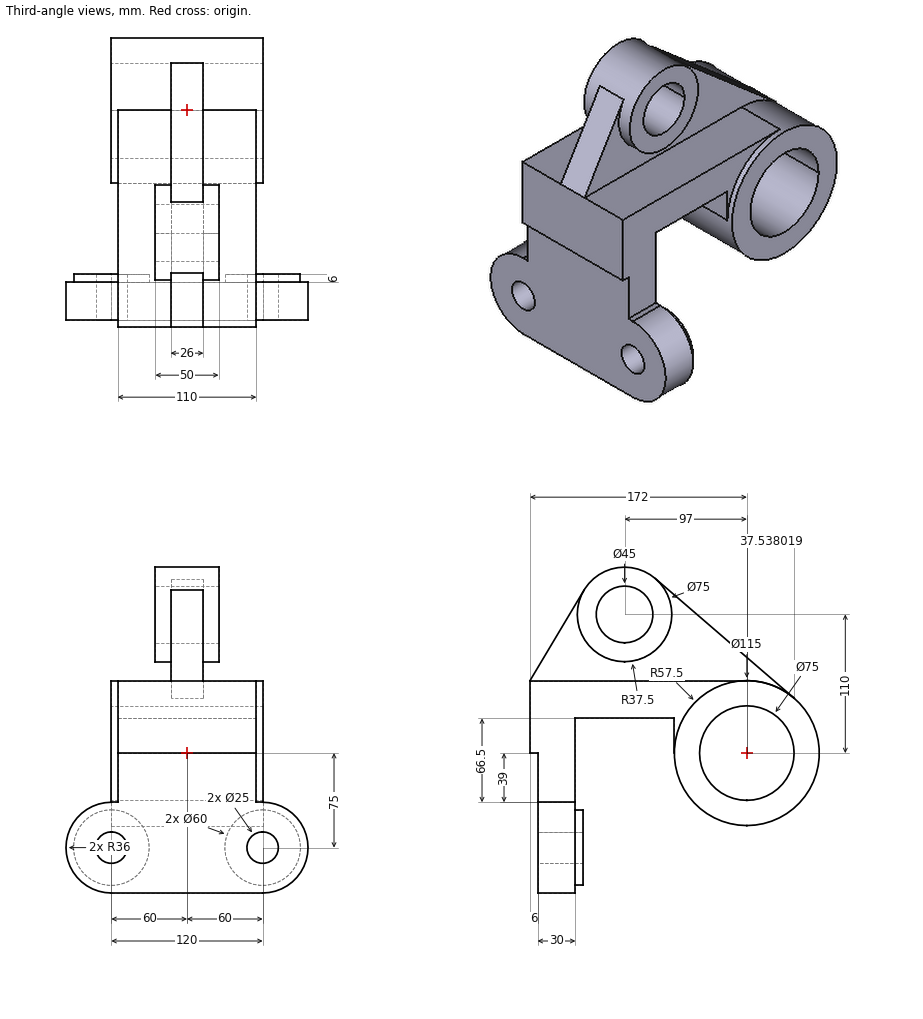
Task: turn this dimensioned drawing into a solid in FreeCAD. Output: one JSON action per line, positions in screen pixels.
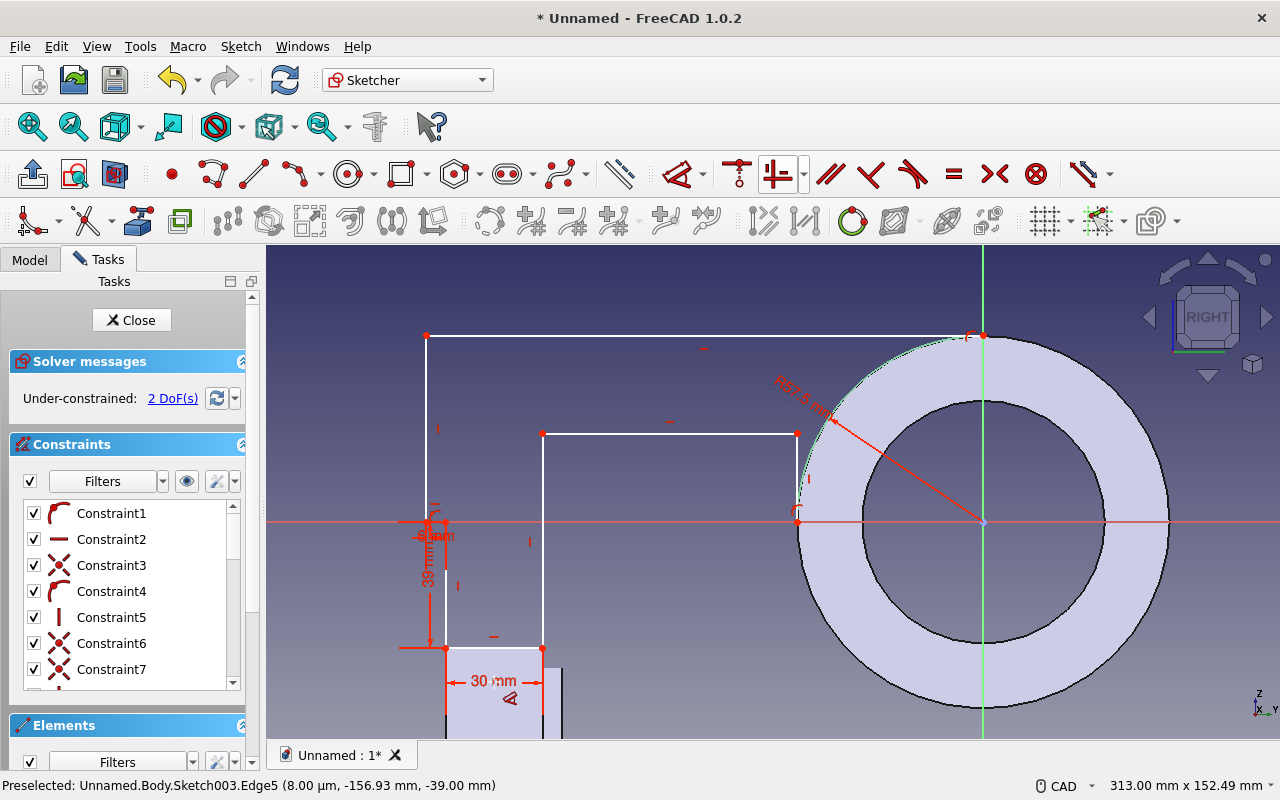
{"action": "left_click", "coordinate": [816, 336]}
{"action": "left_click", "coordinate": [705, 302]}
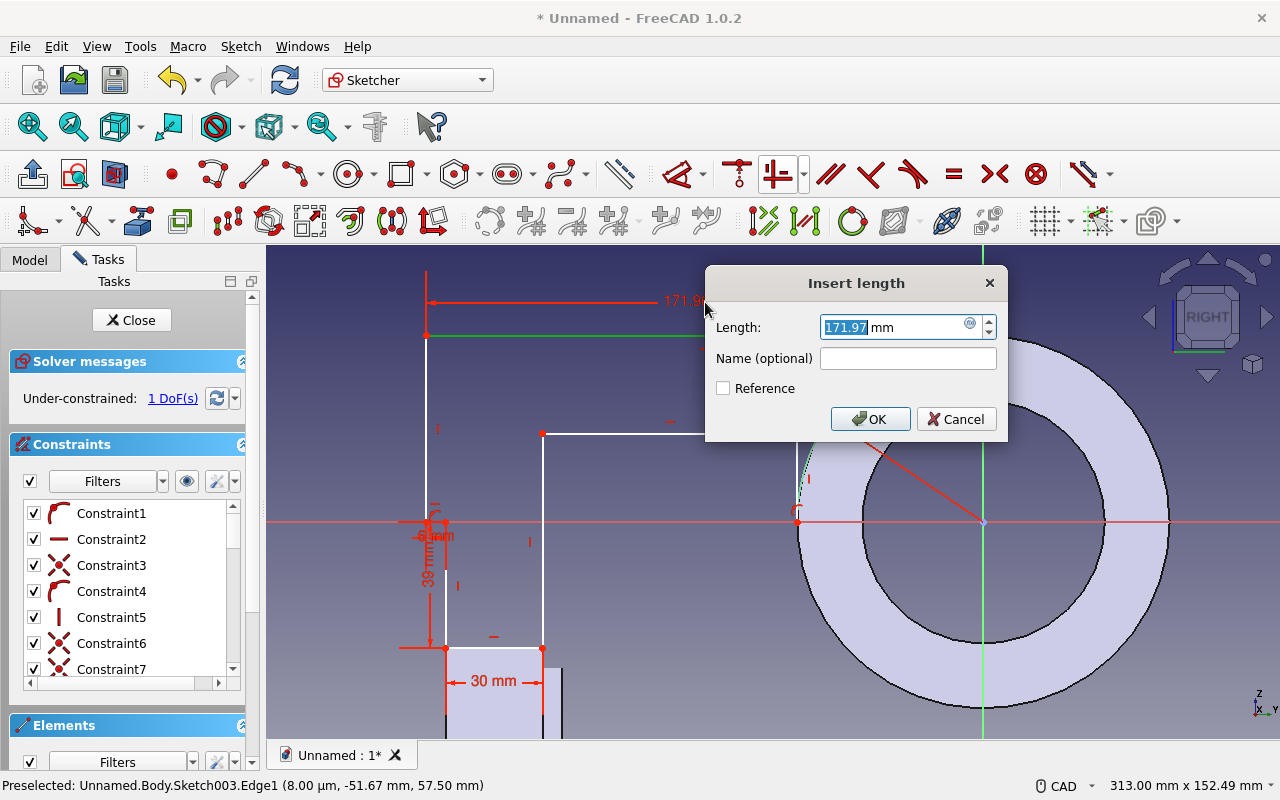
{"action": "type", "text": "172"}
{"action": "key", "text": "Return"}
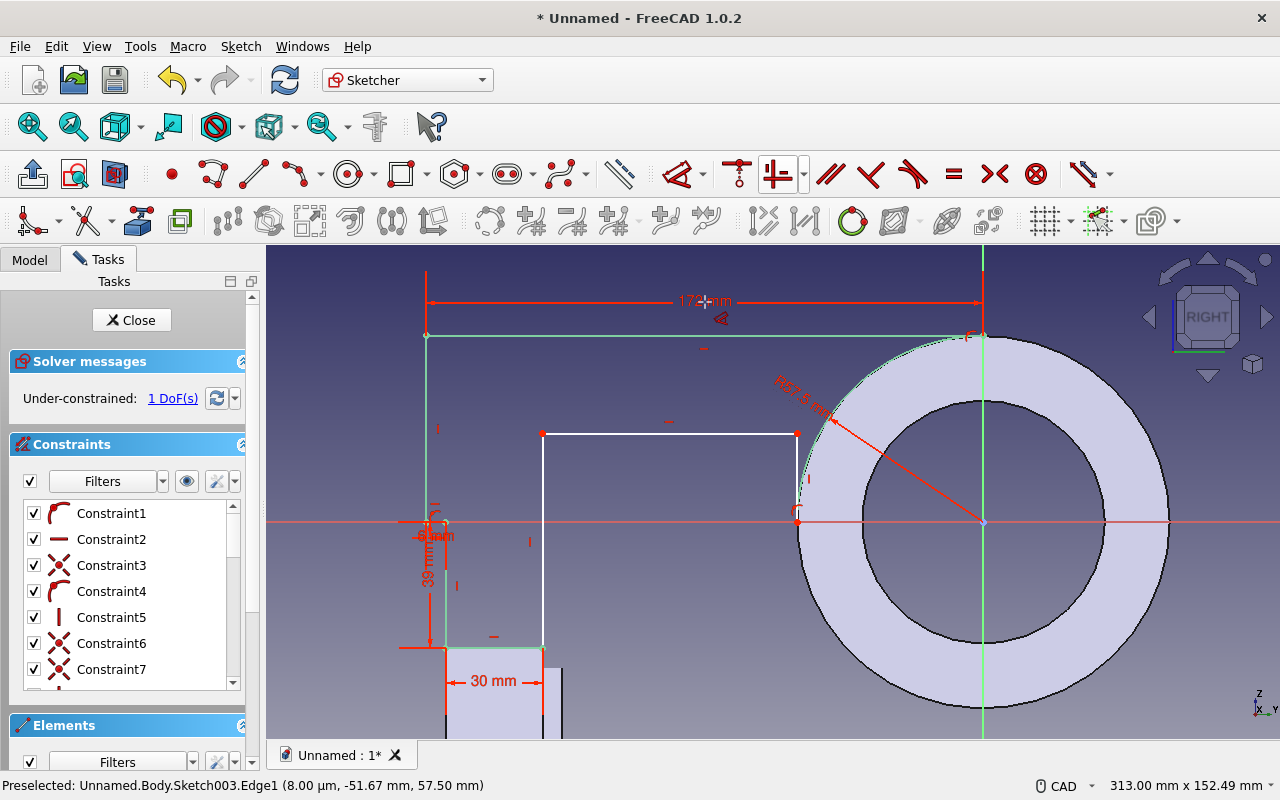
{"action": "left_click", "coordinate": [543, 584]}
{"action": "left_click", "coordinate": [509, 541]}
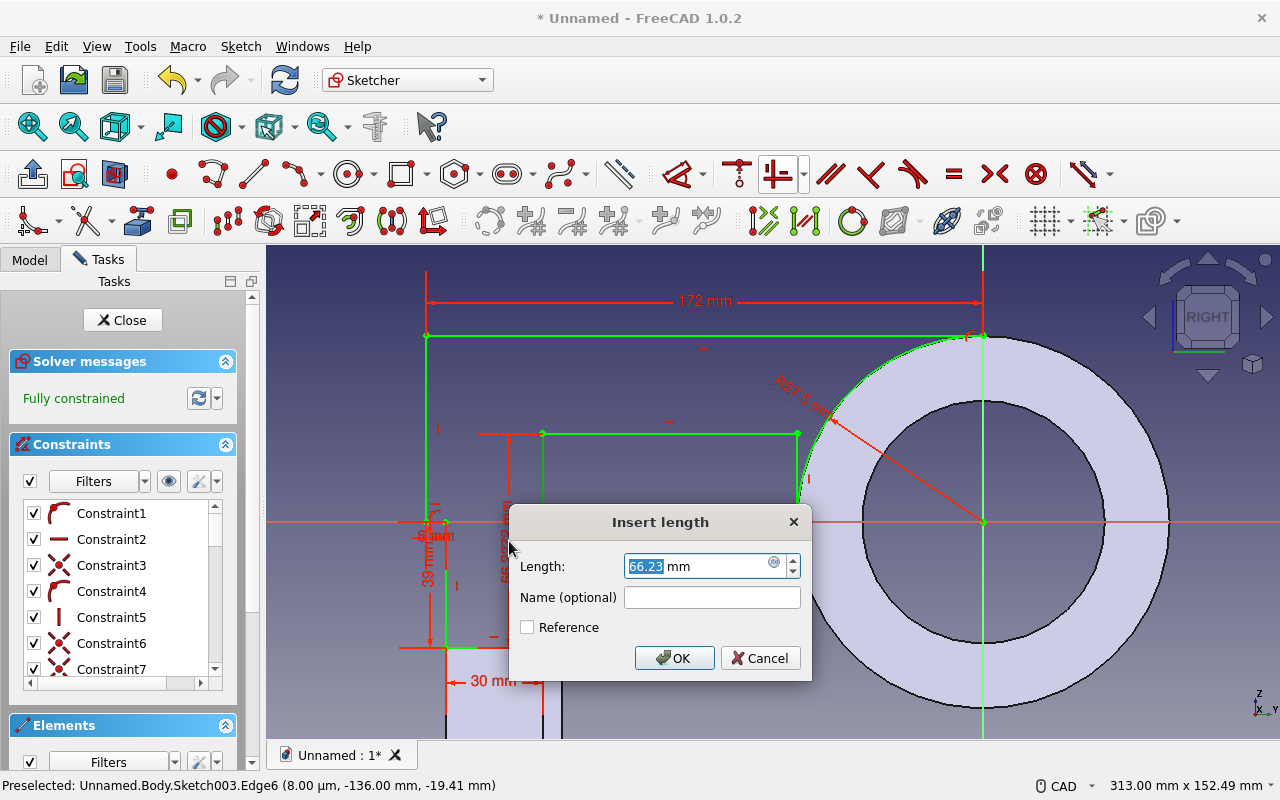
{"action": "type", "text": "66.5"}
{"action": "key", "text": "Return"}
{"action": "key", "text": "Escape"}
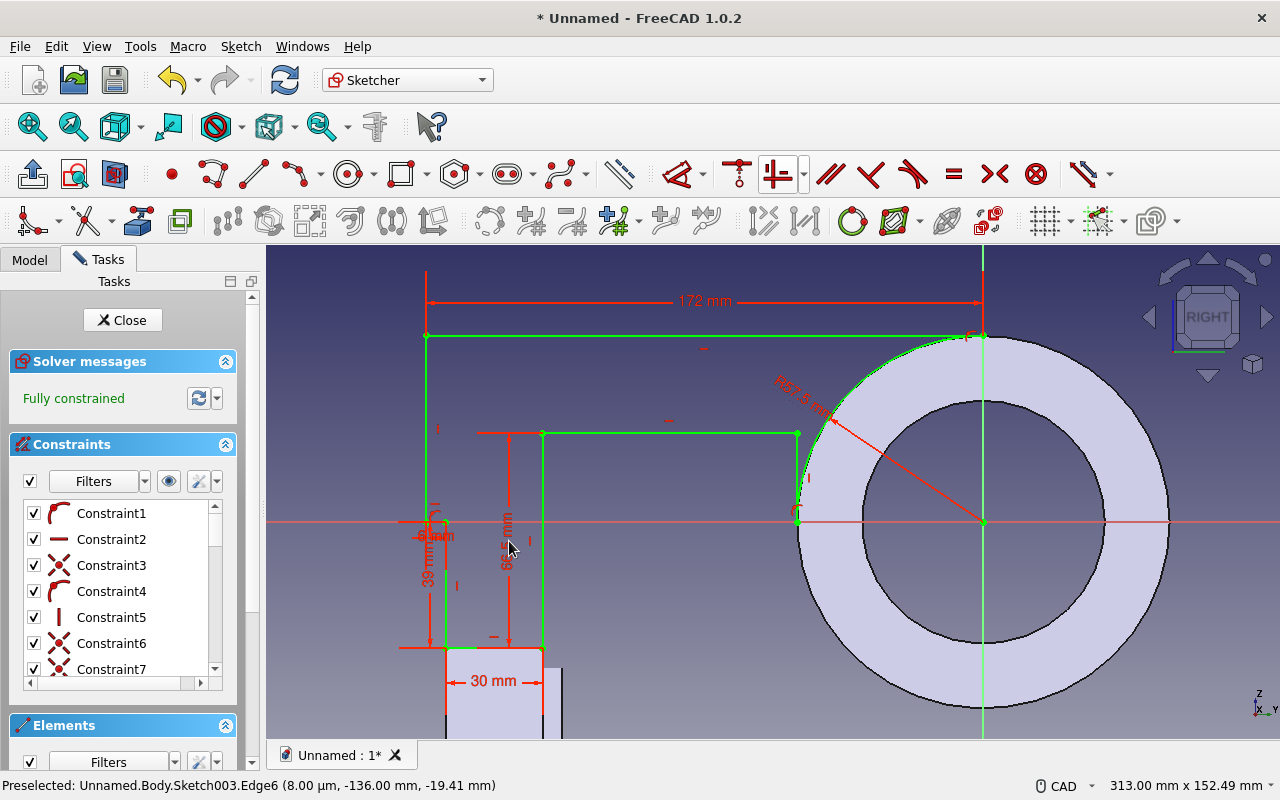
{"action": "left_click", "coordinate": [123, 320]}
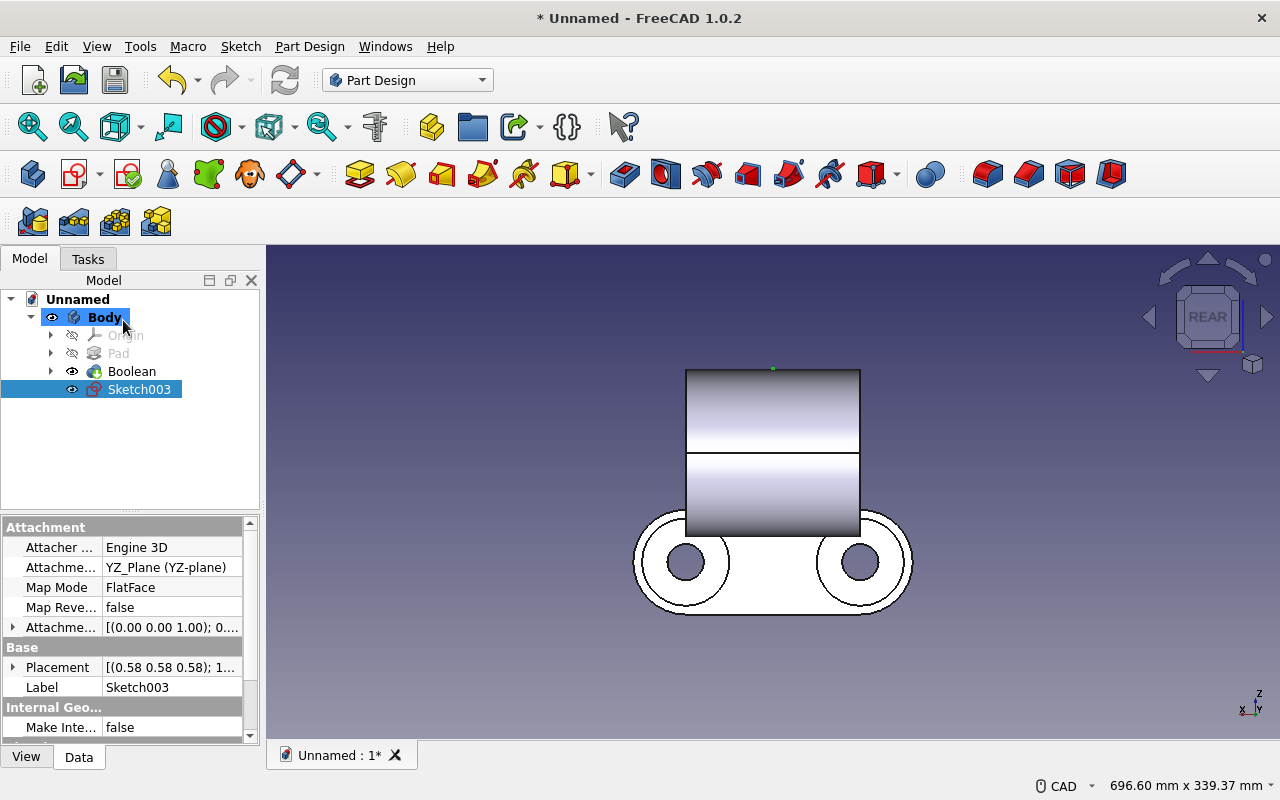
{"action": "left_click", "coordinate": [360, 174]}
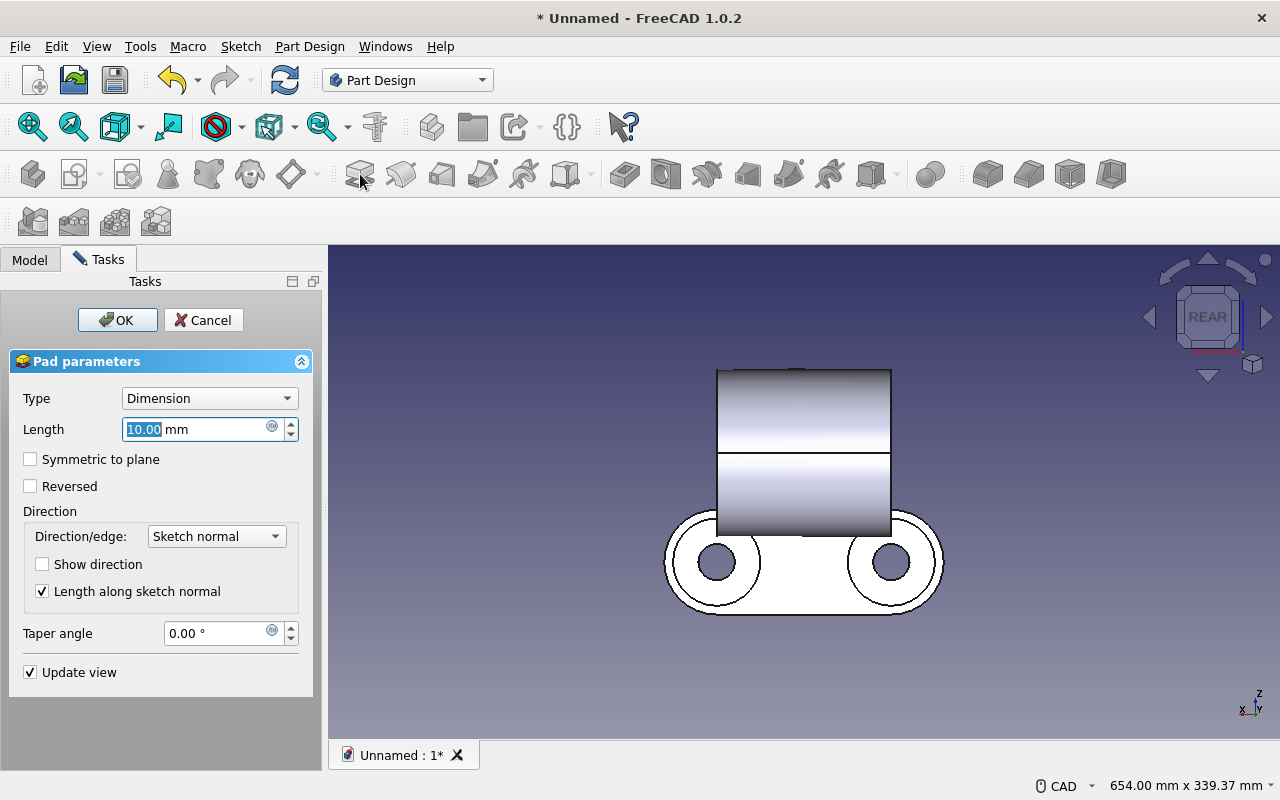
{"action": "type", "text": "110"}
{"action": "key", "text": "Tab"}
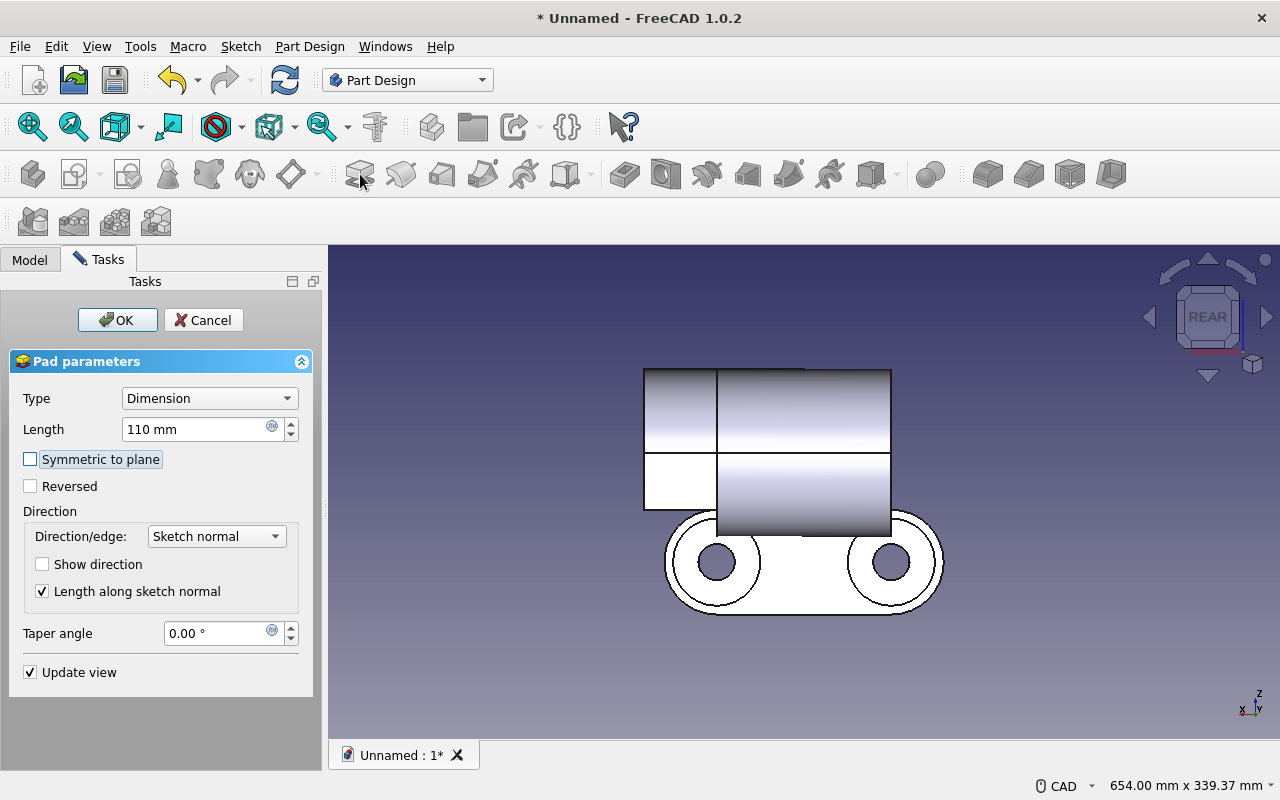
{"action": "left_click", "coordinate": [31, 459]}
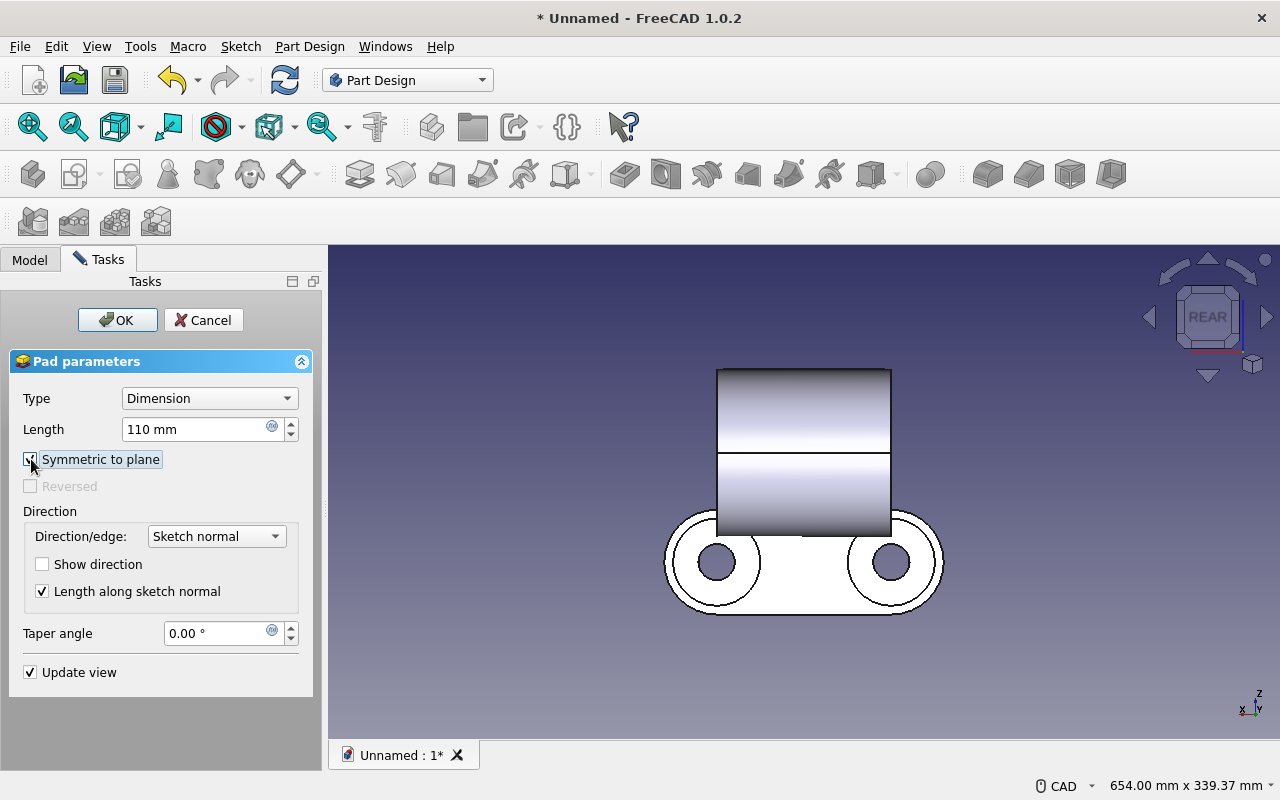
{"action": "left_click", "coordinate": [118, 320]}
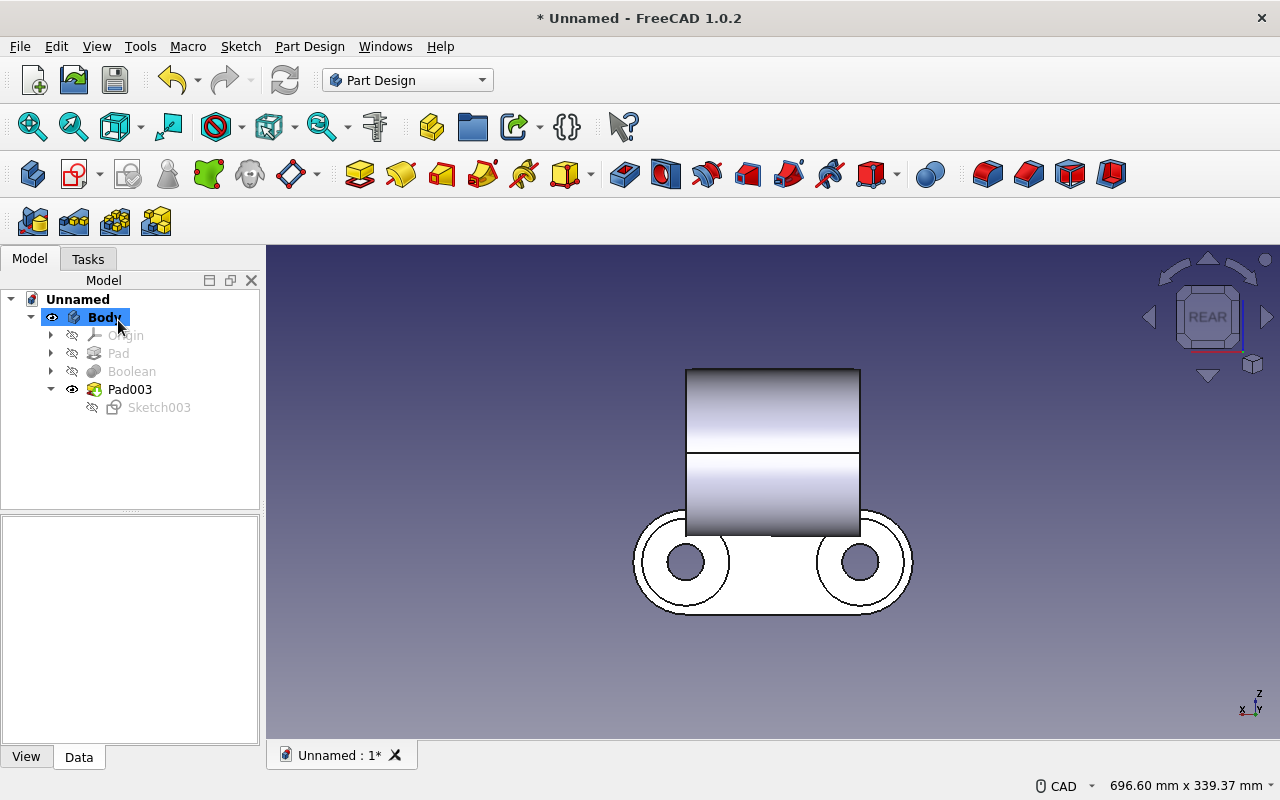
{"action": "left_click", "coordinate": [33, 174]}